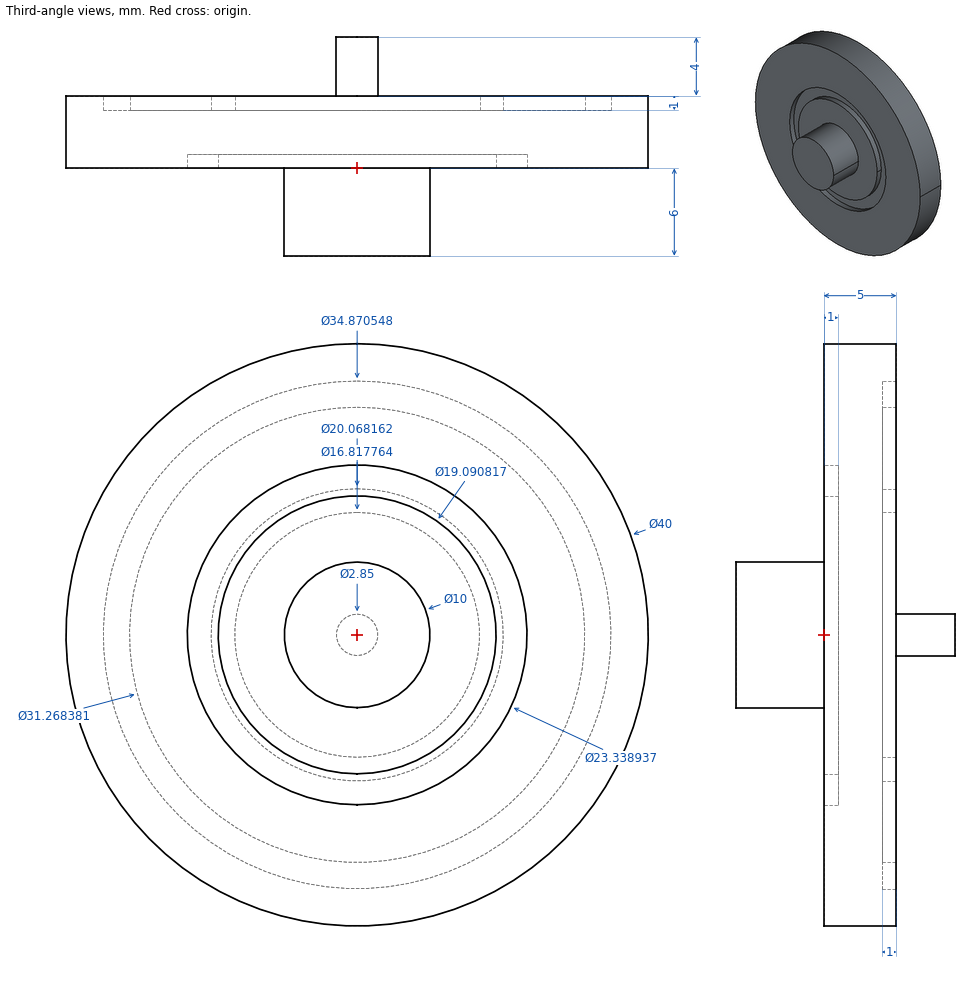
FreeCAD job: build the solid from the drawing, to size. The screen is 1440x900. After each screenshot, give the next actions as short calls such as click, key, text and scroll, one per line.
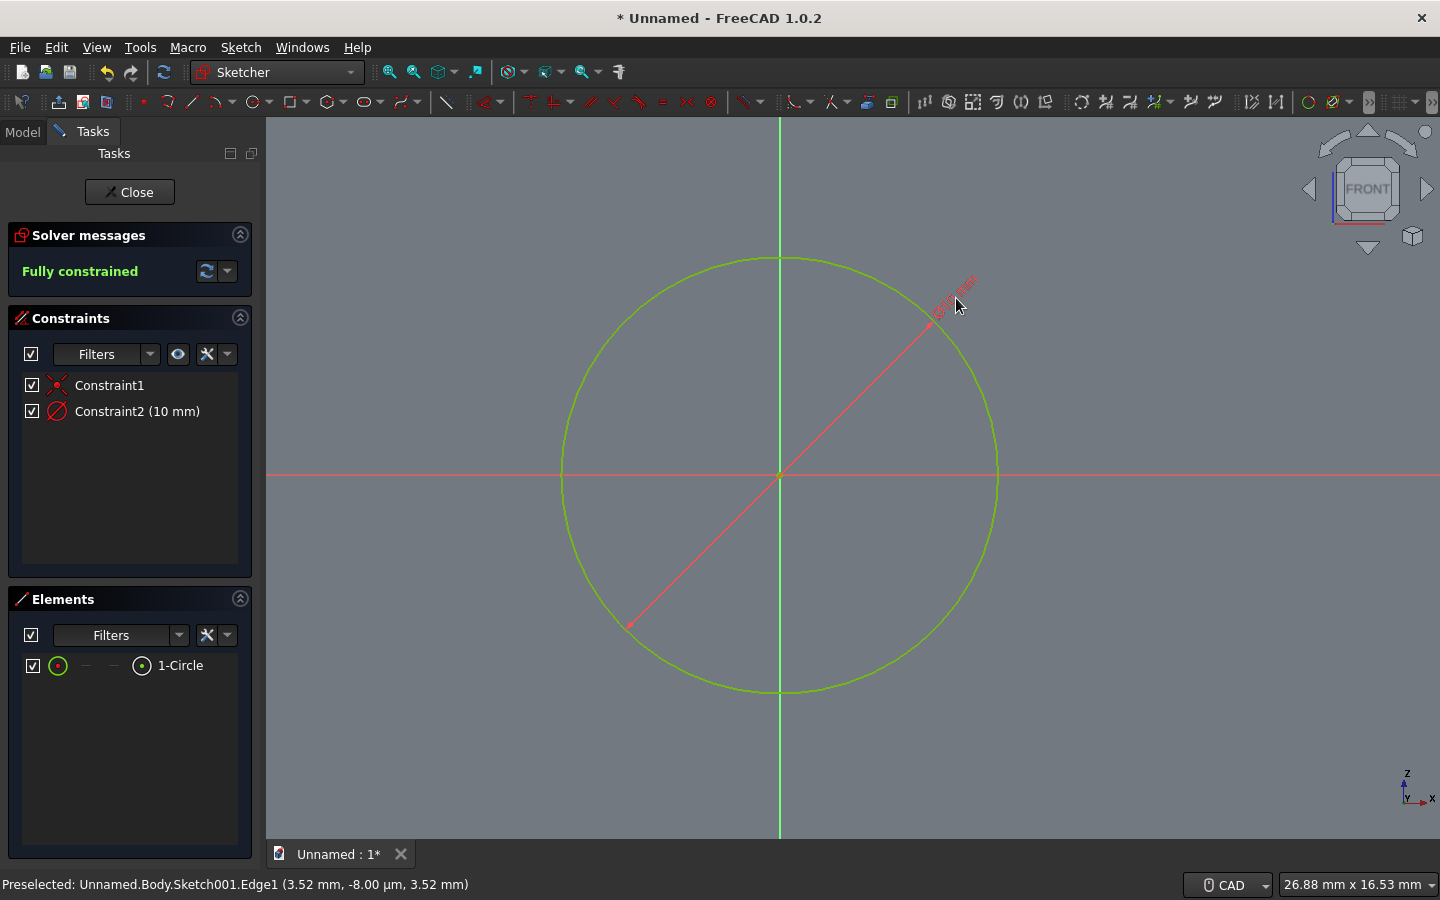
click(130, 192)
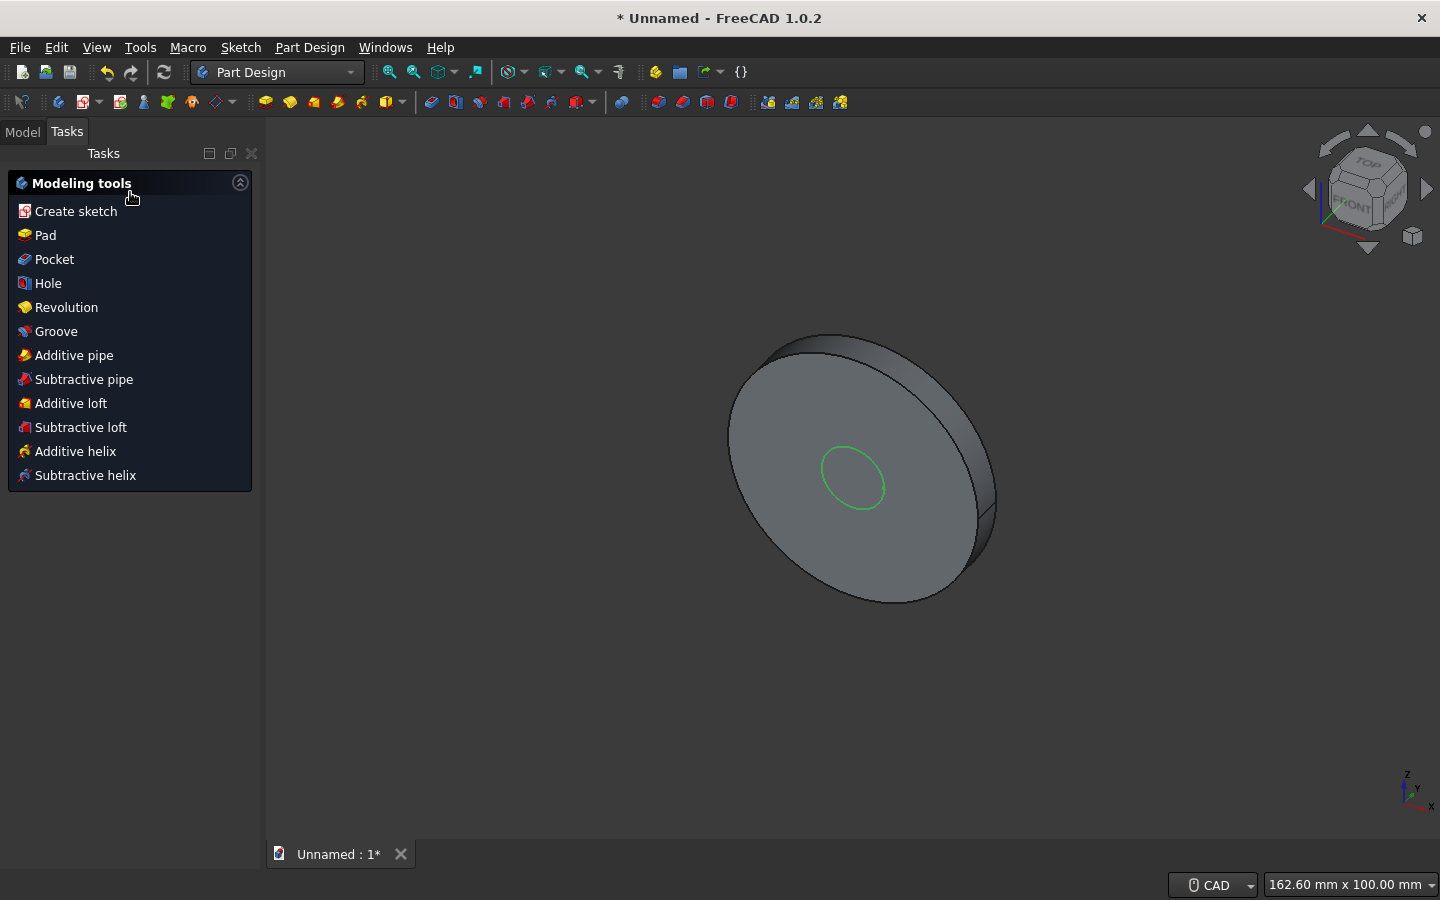
click(266, 102)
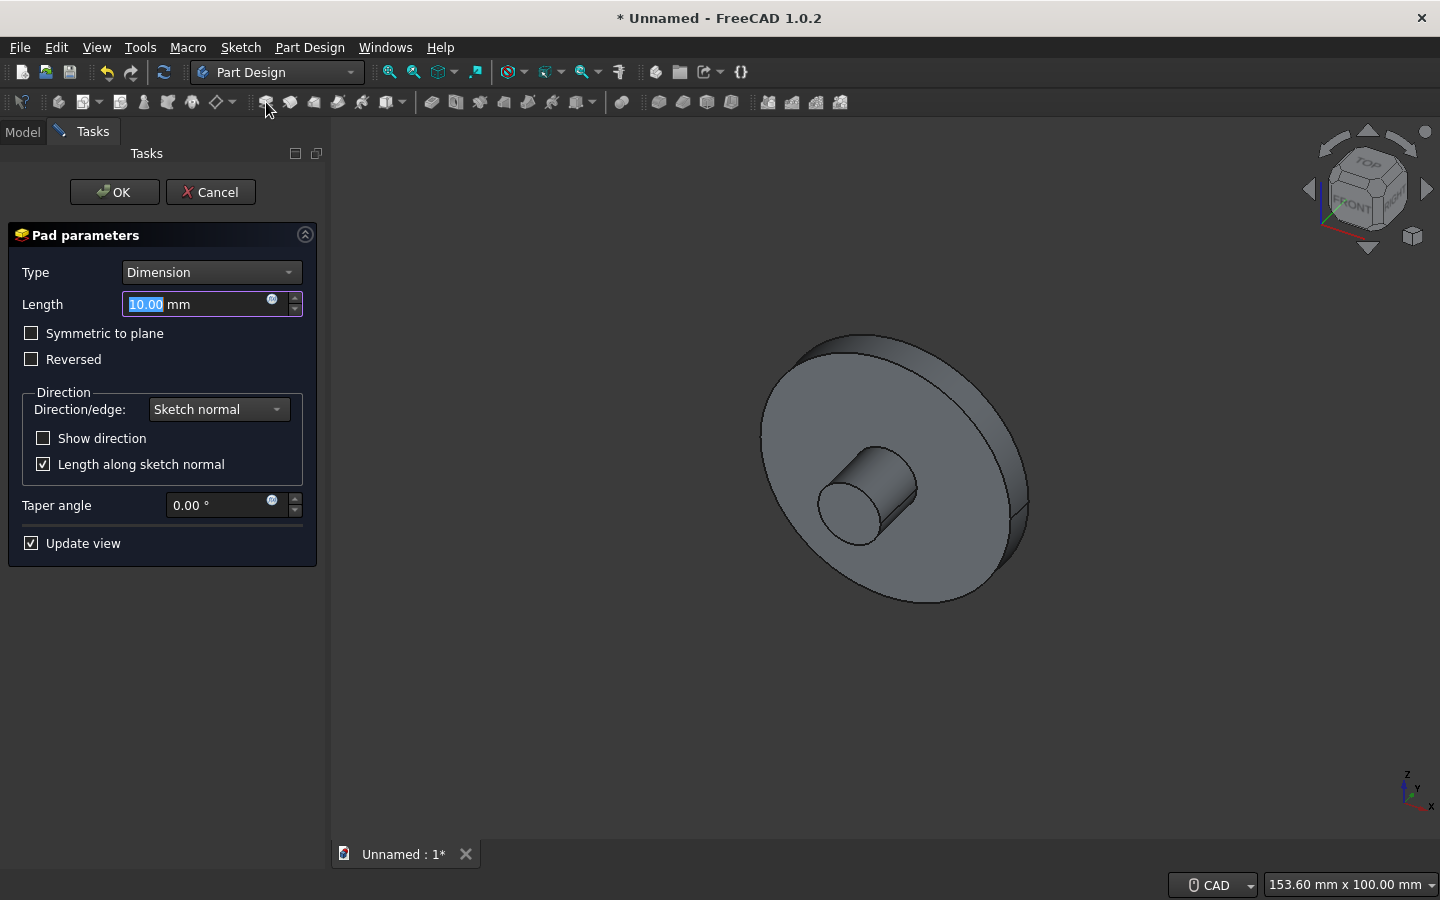
text(6)
key(Tab)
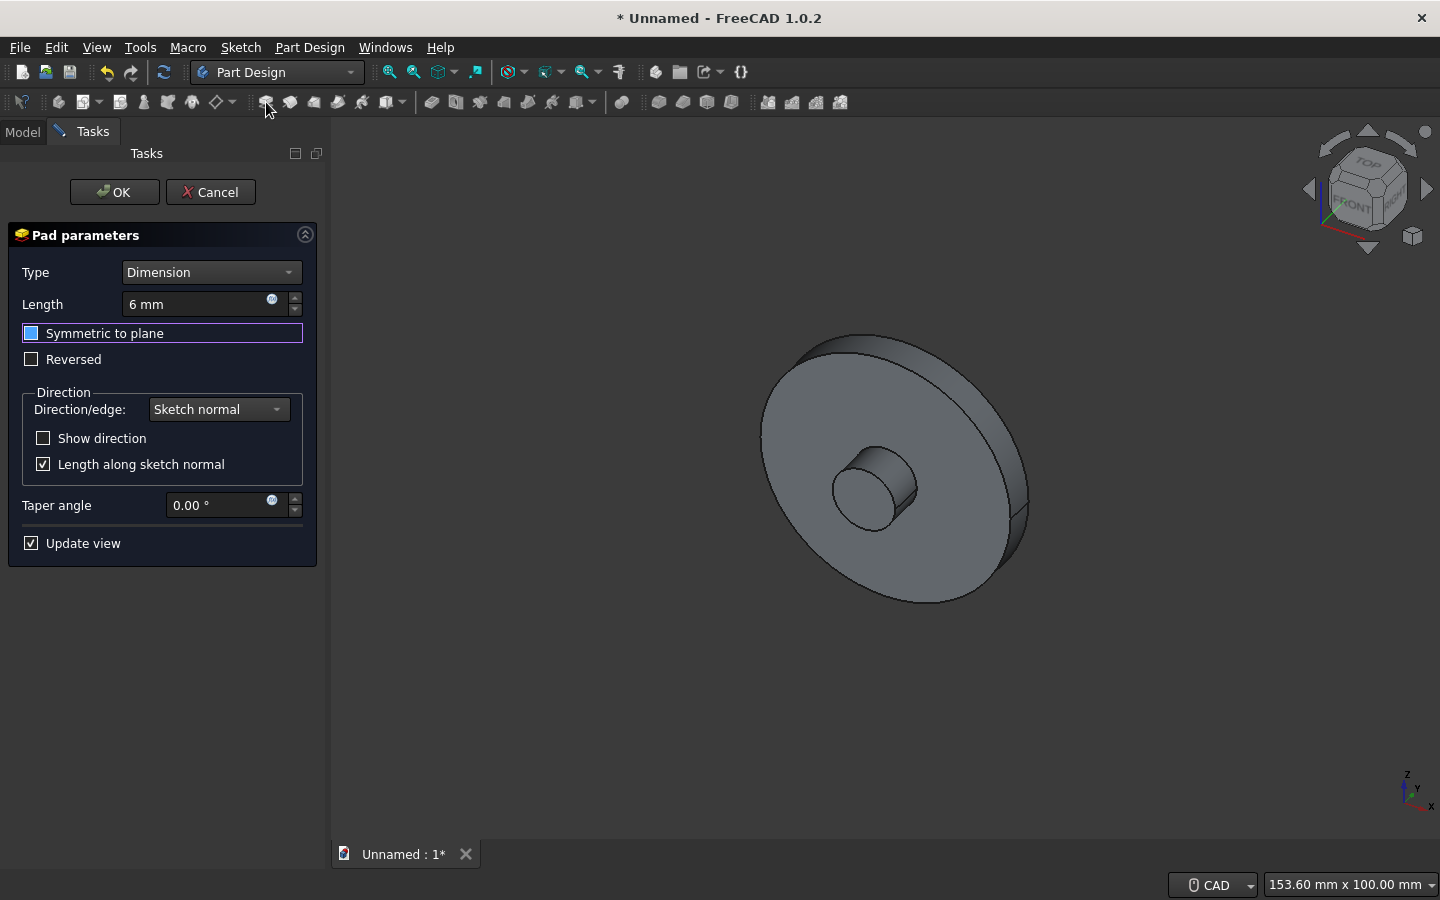
click(115, 192)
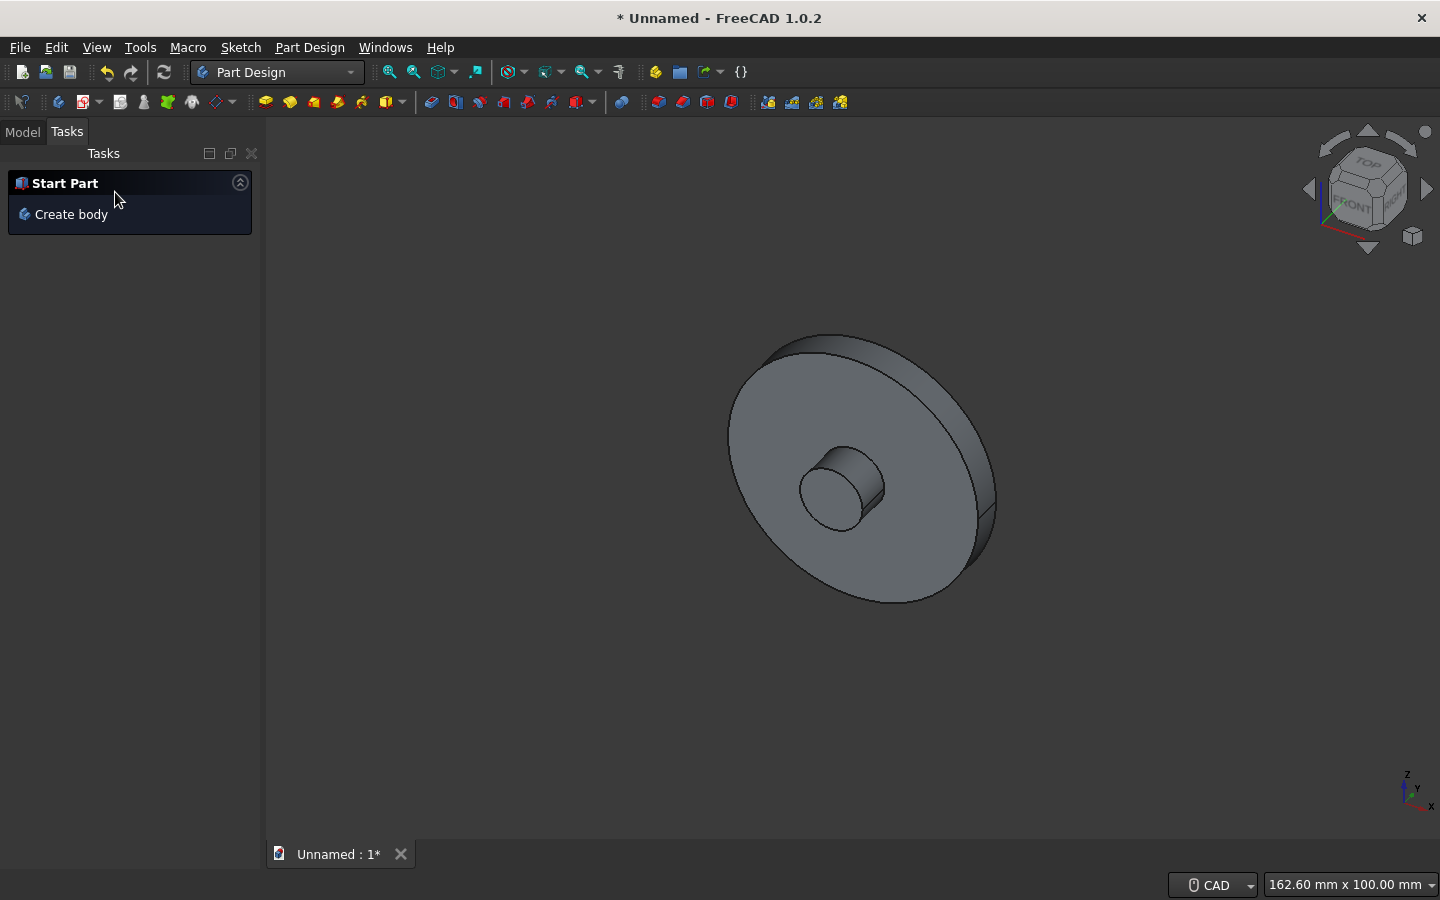
click(84, 102)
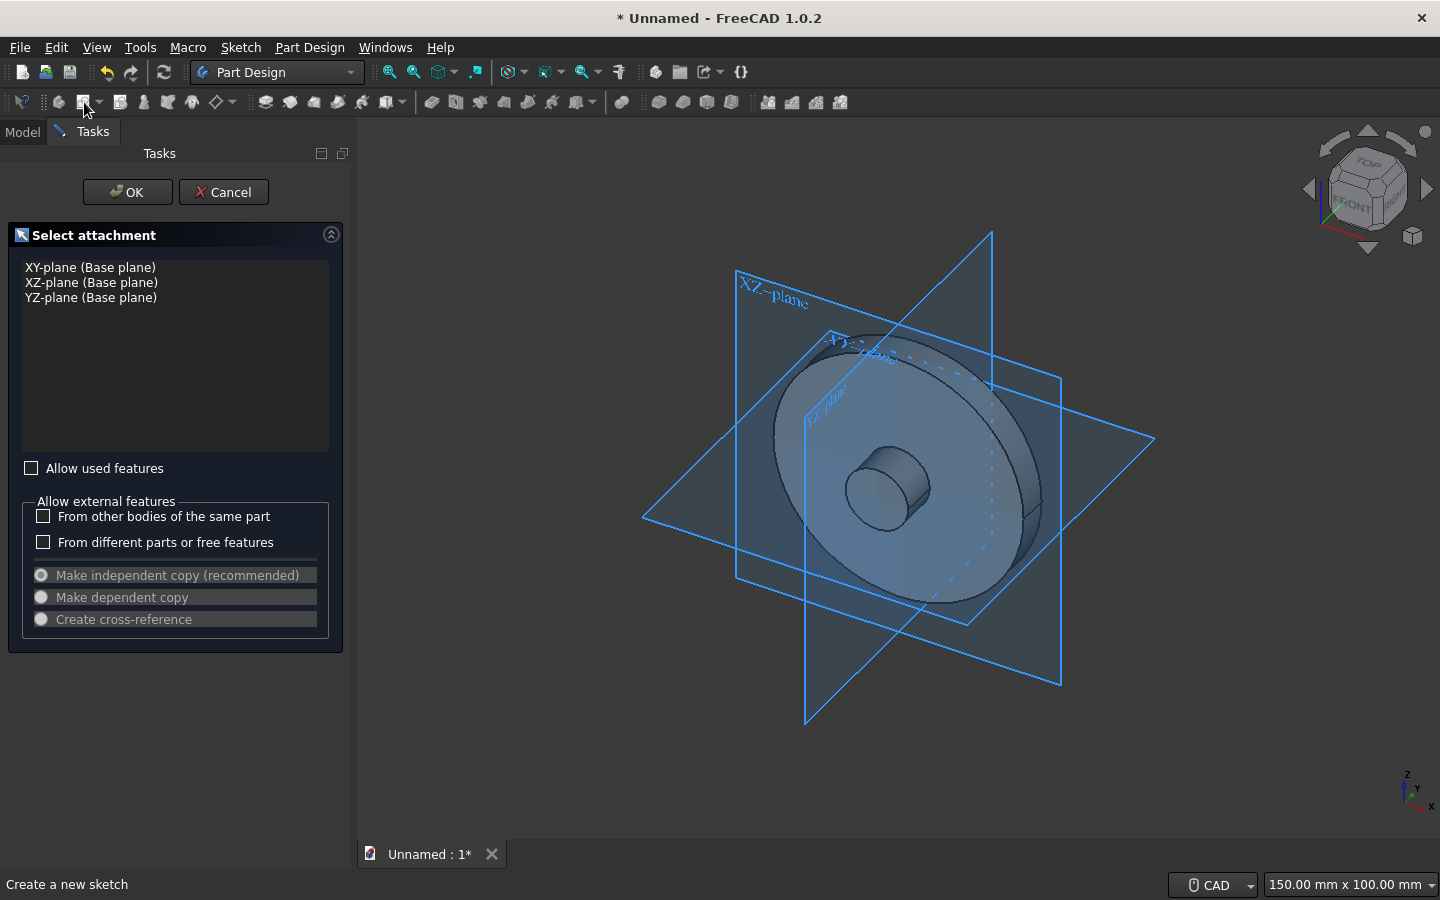
click(82, 282)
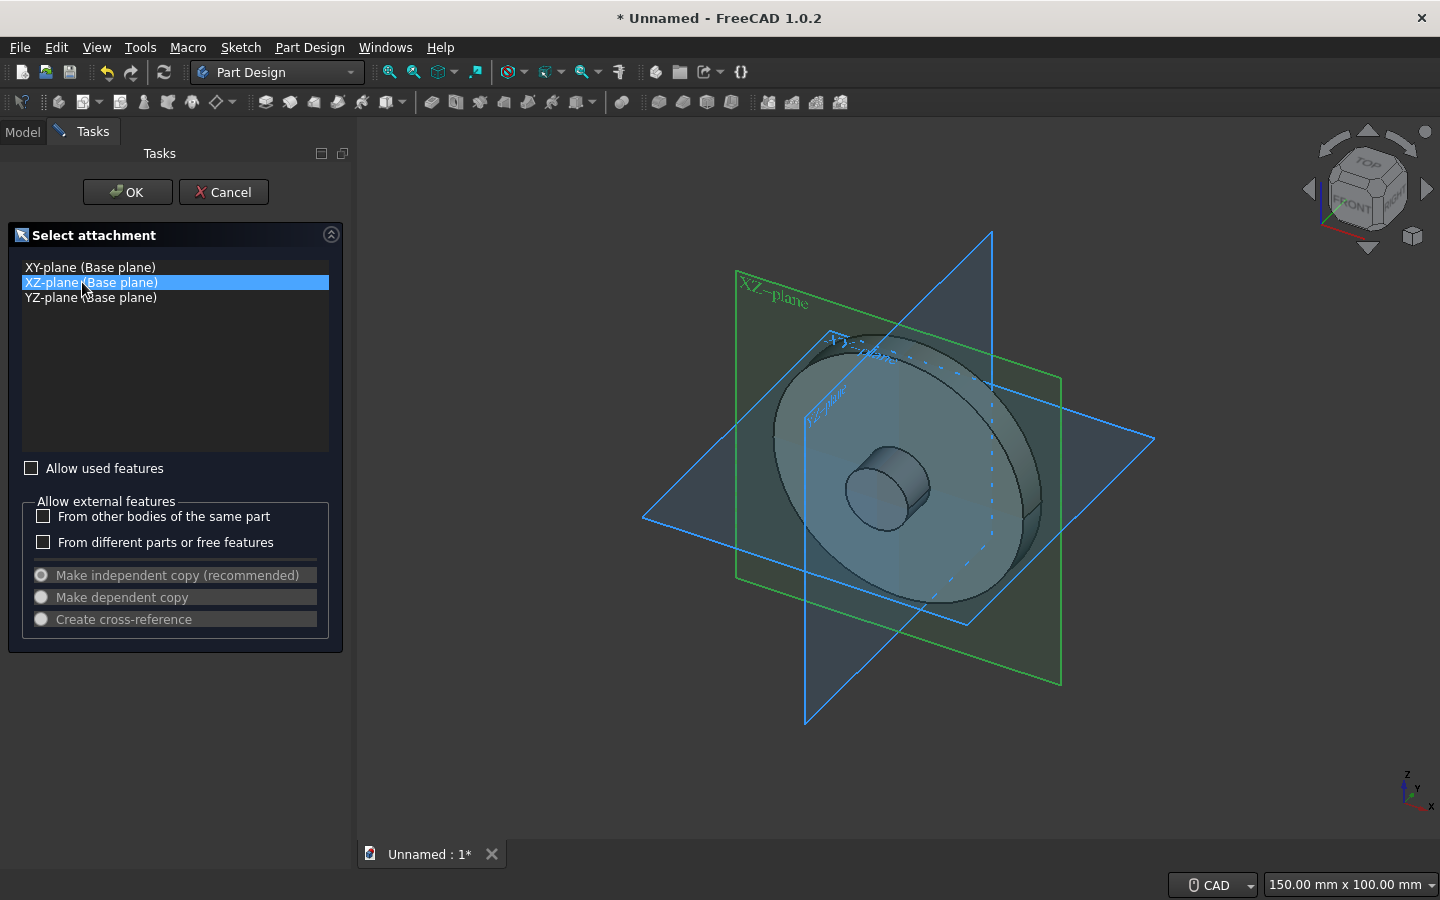
click(128, 192)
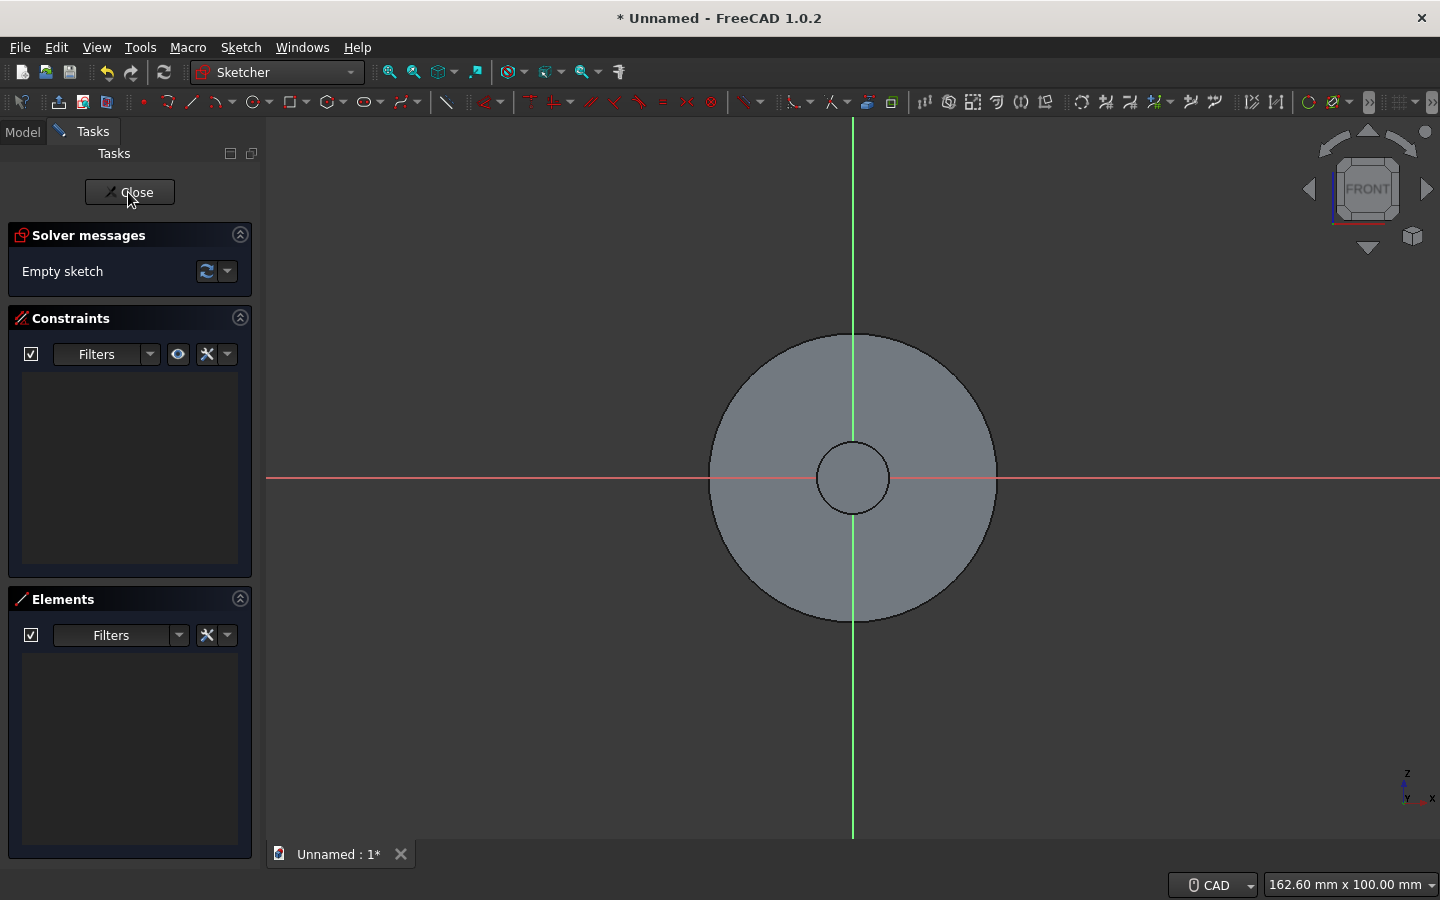
key(q)
key(s)